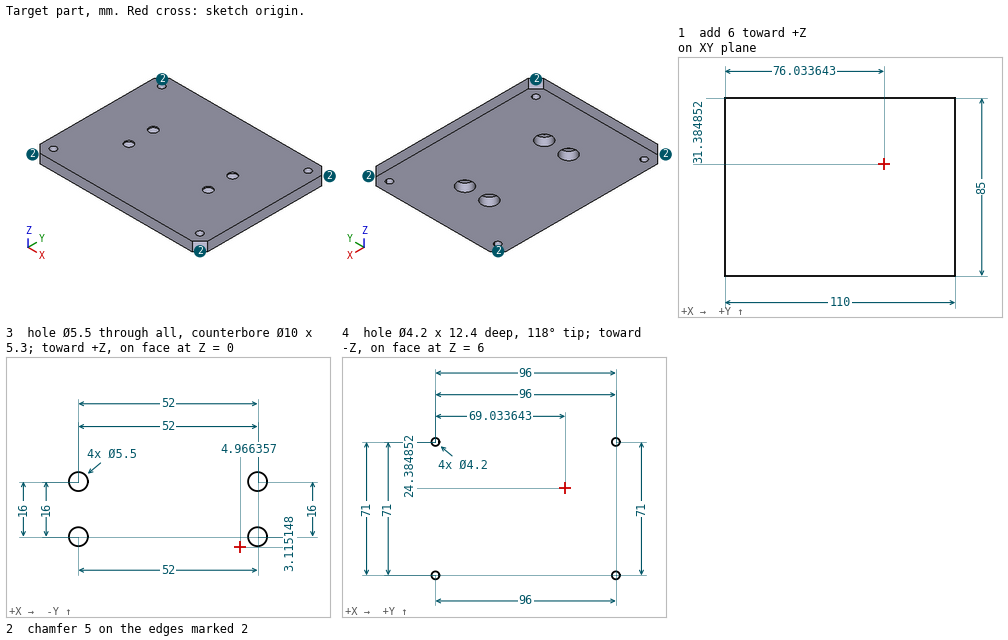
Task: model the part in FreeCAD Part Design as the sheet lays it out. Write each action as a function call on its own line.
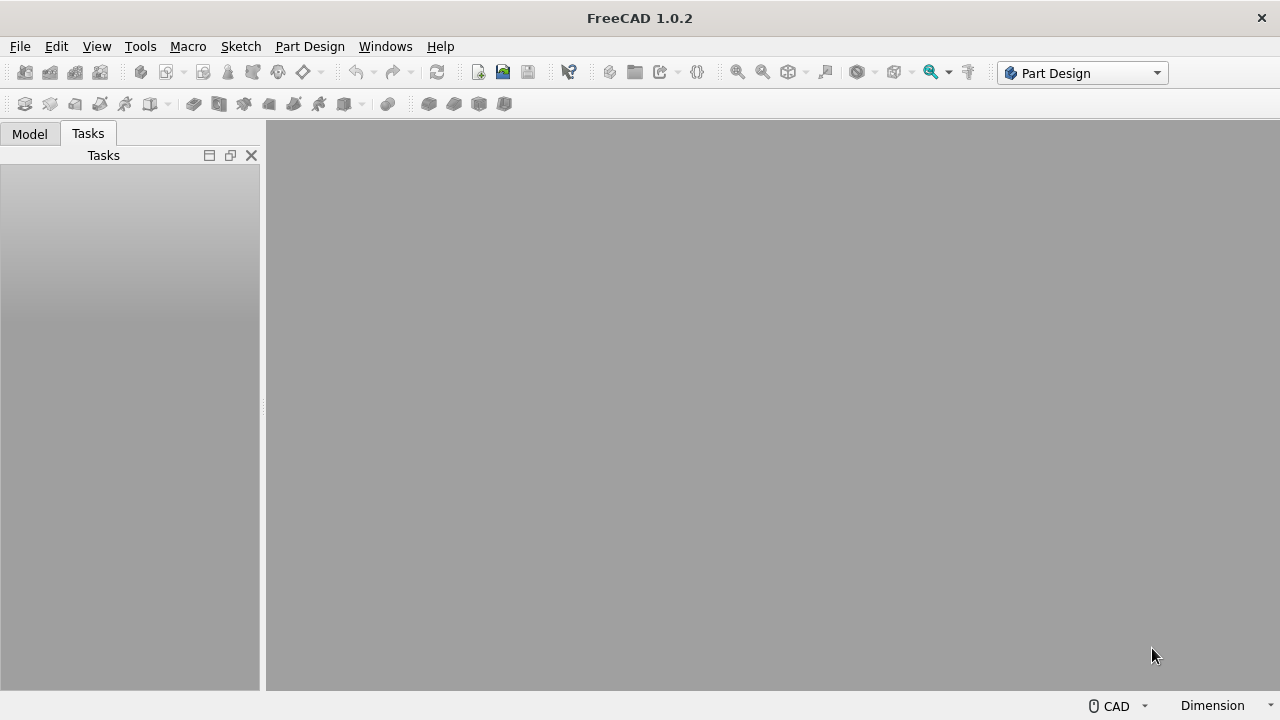
click(478, 72)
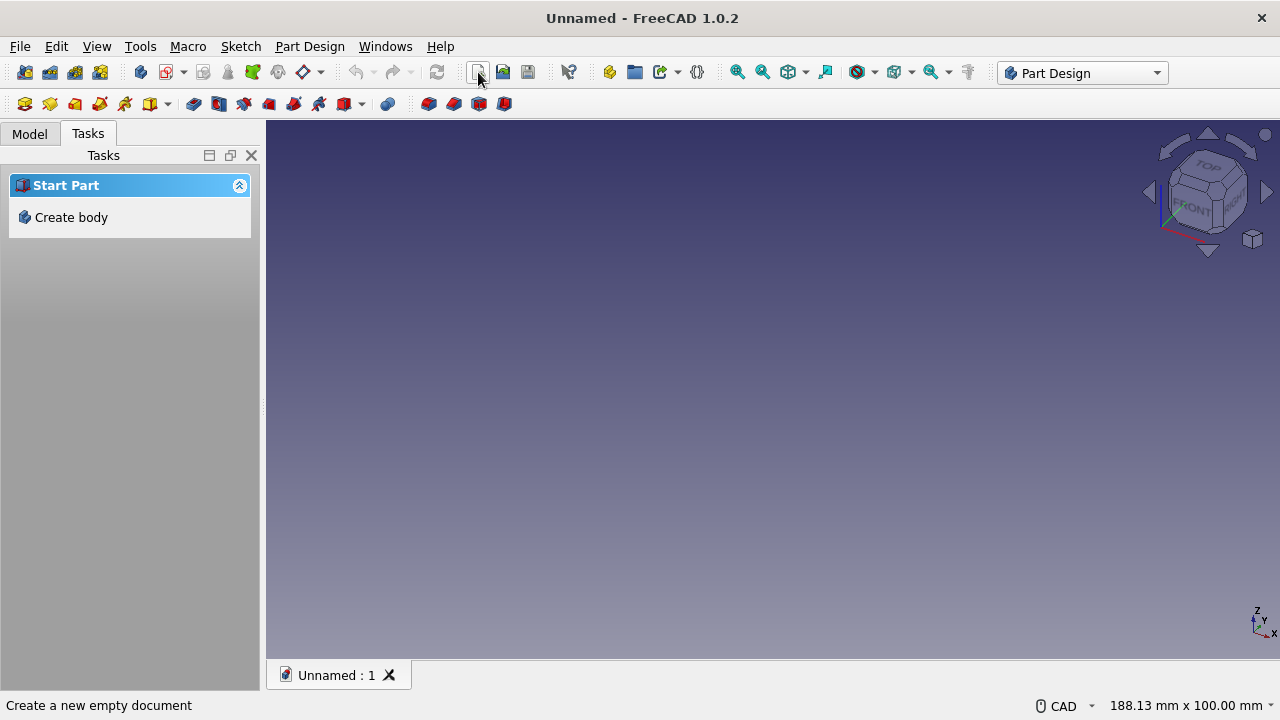
click(166, 72)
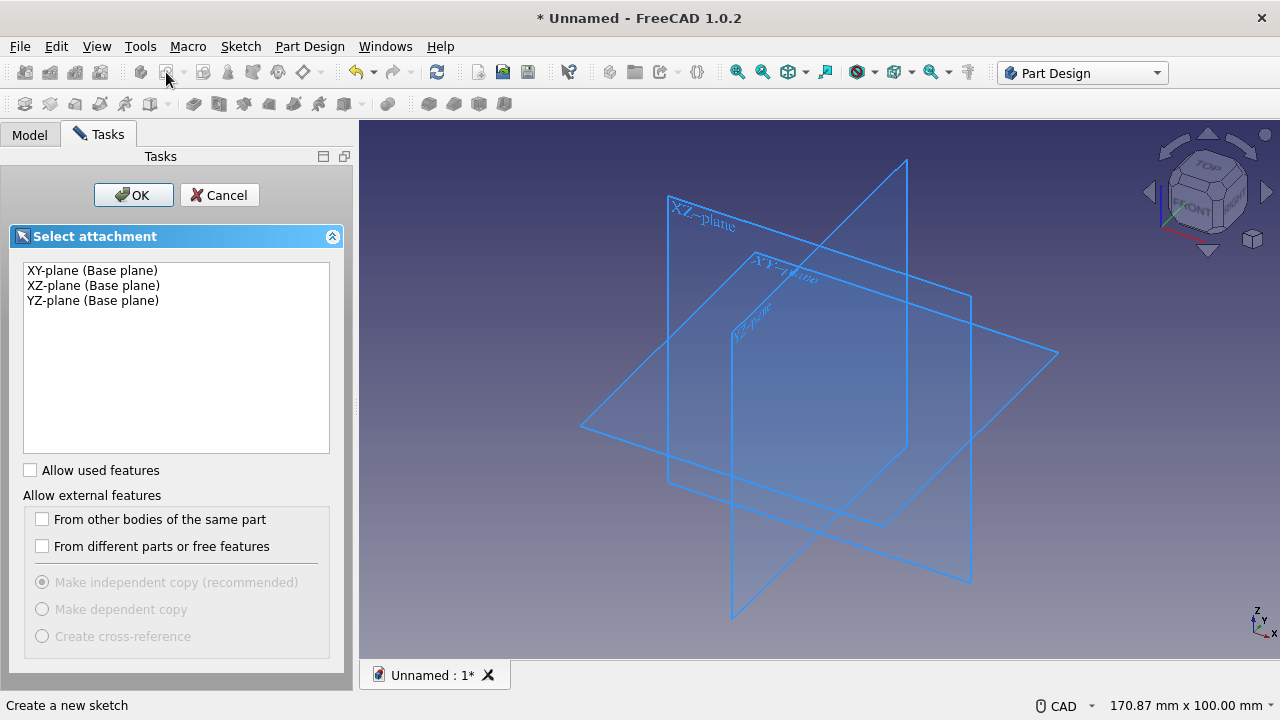
click(84, 270)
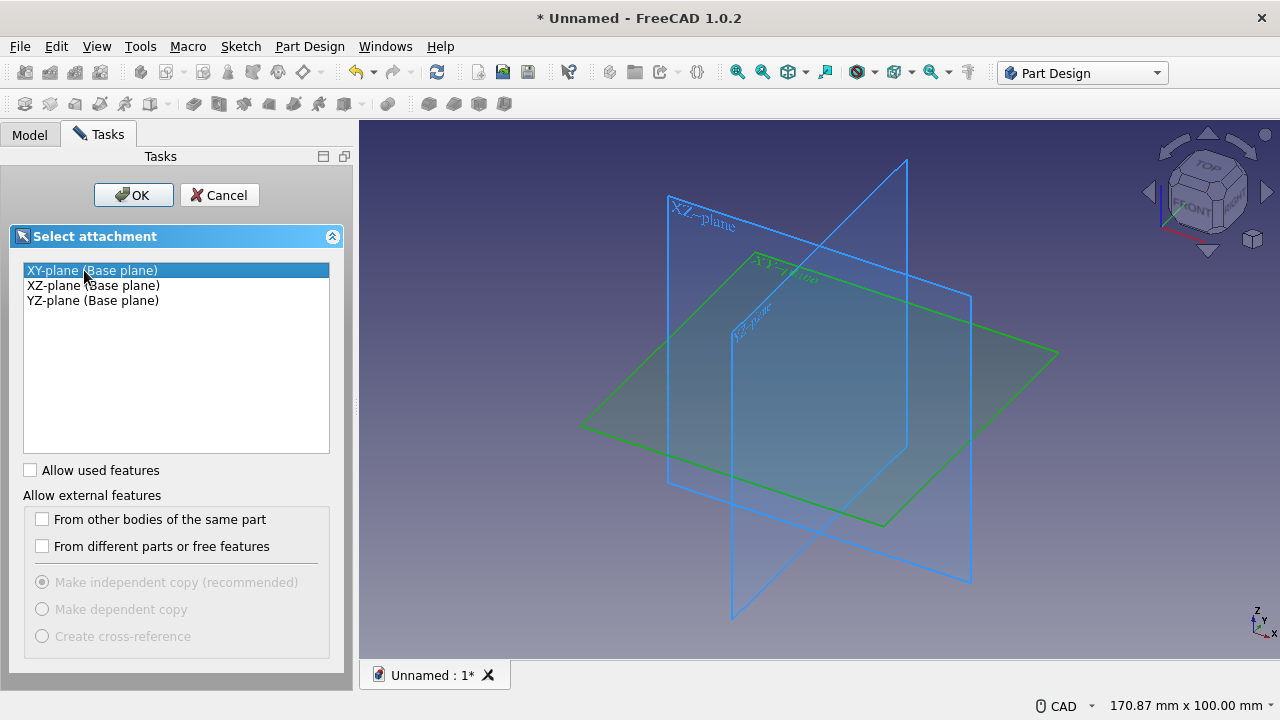
click(134, 195)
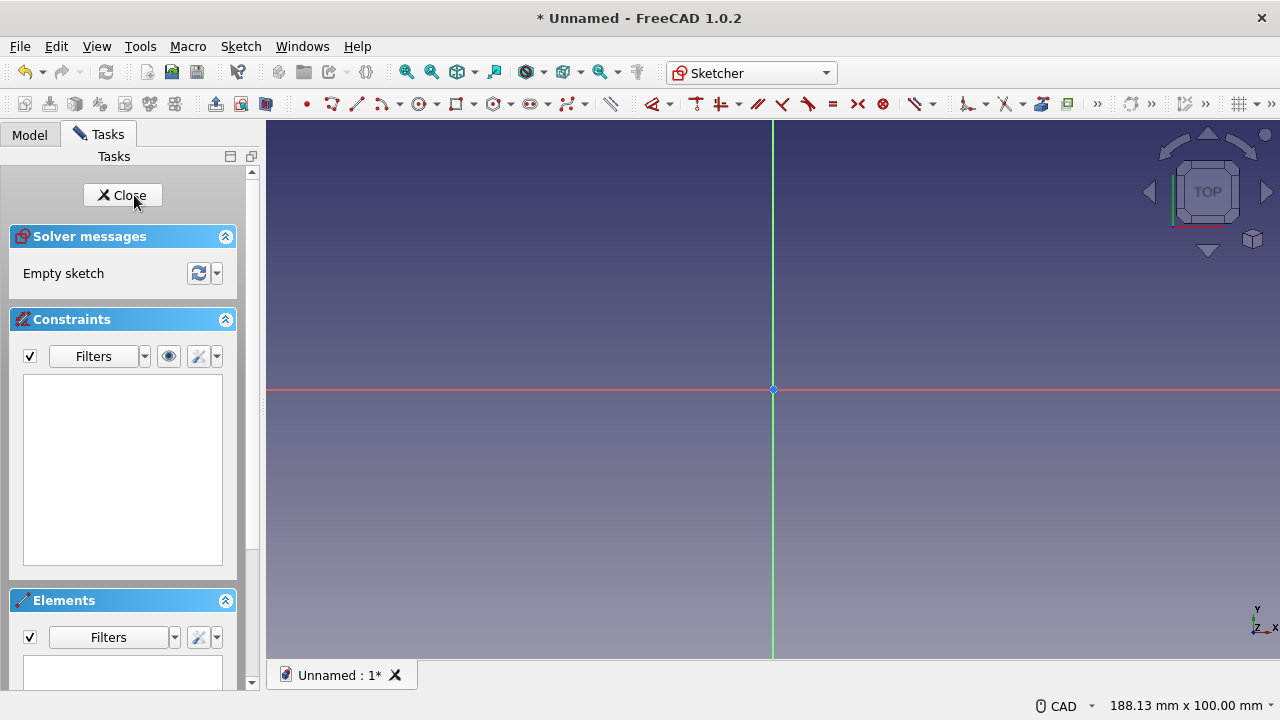
scroll(907, 148, down, 1)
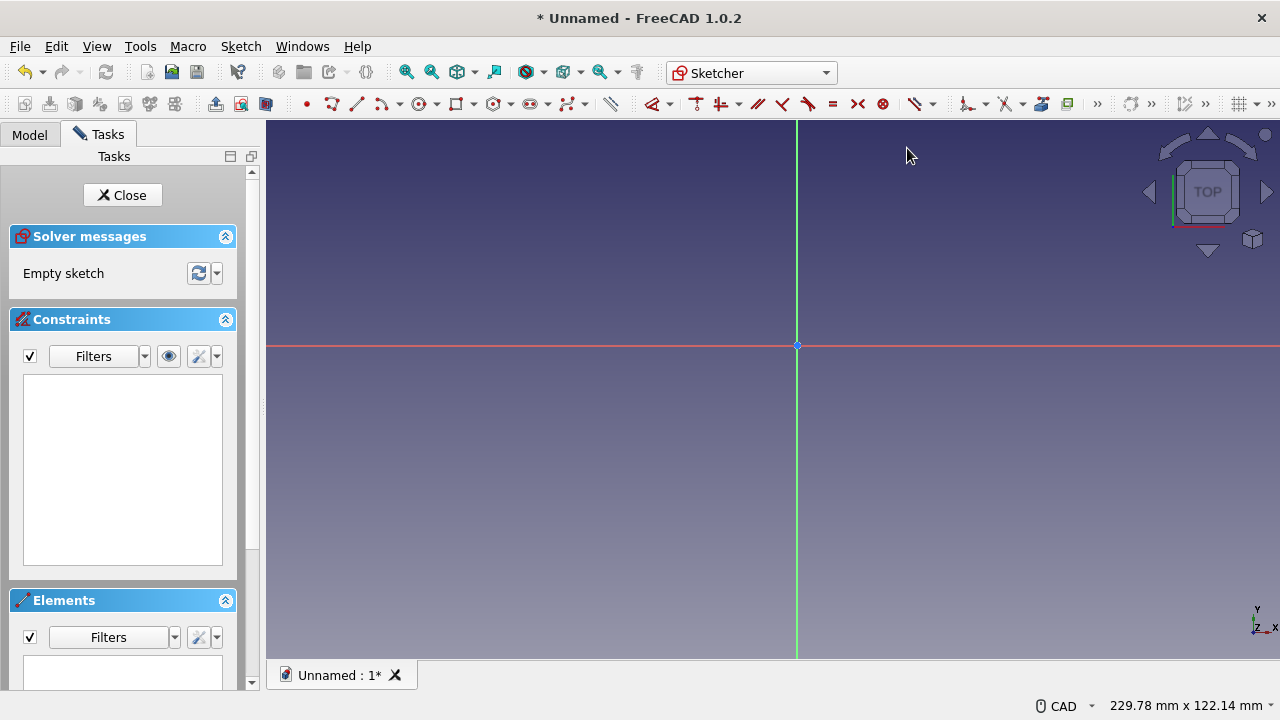
key(g)
key(r)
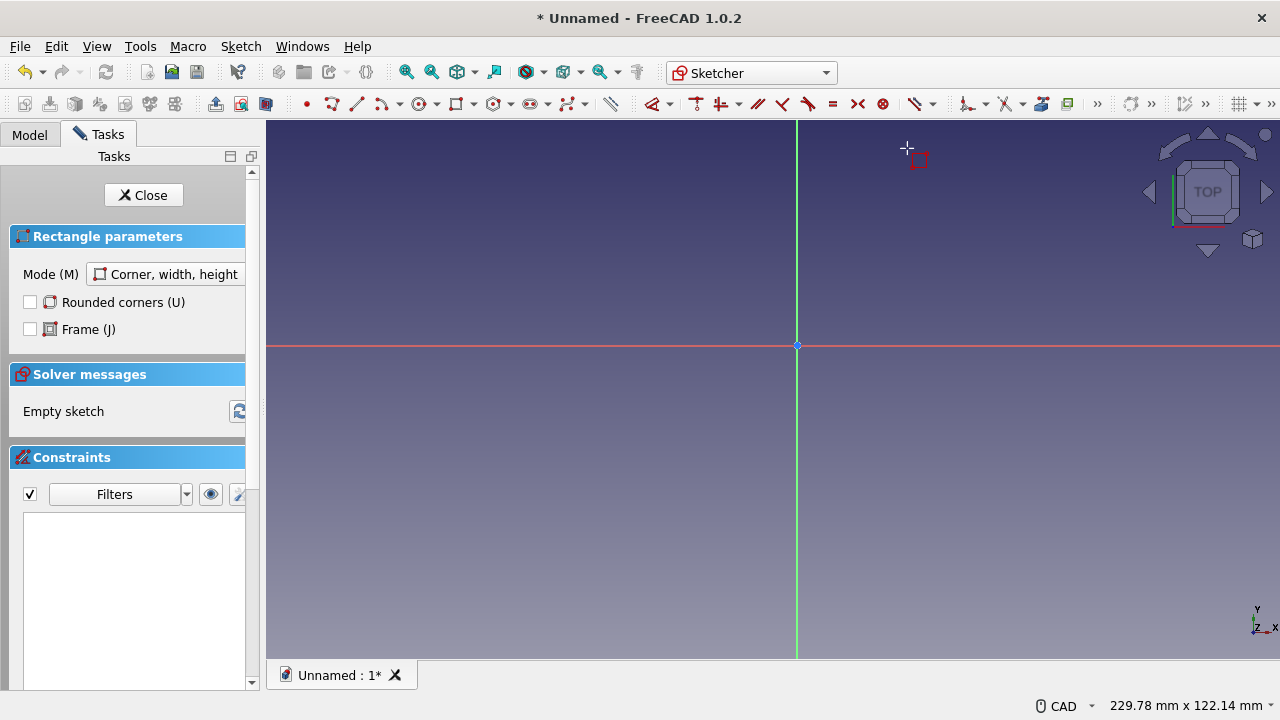
click(462, 207)
move(947, 582)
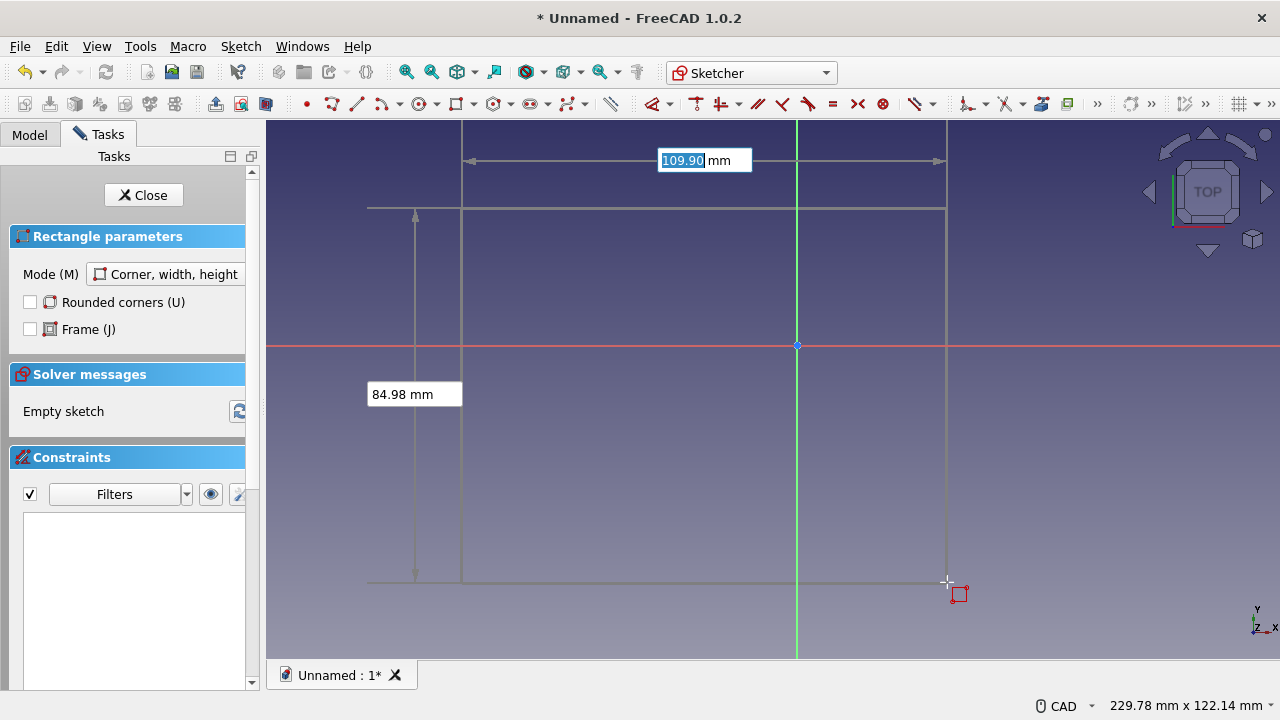
text(110)
key(Tab)
text(85)
key(Return)
key(Escape)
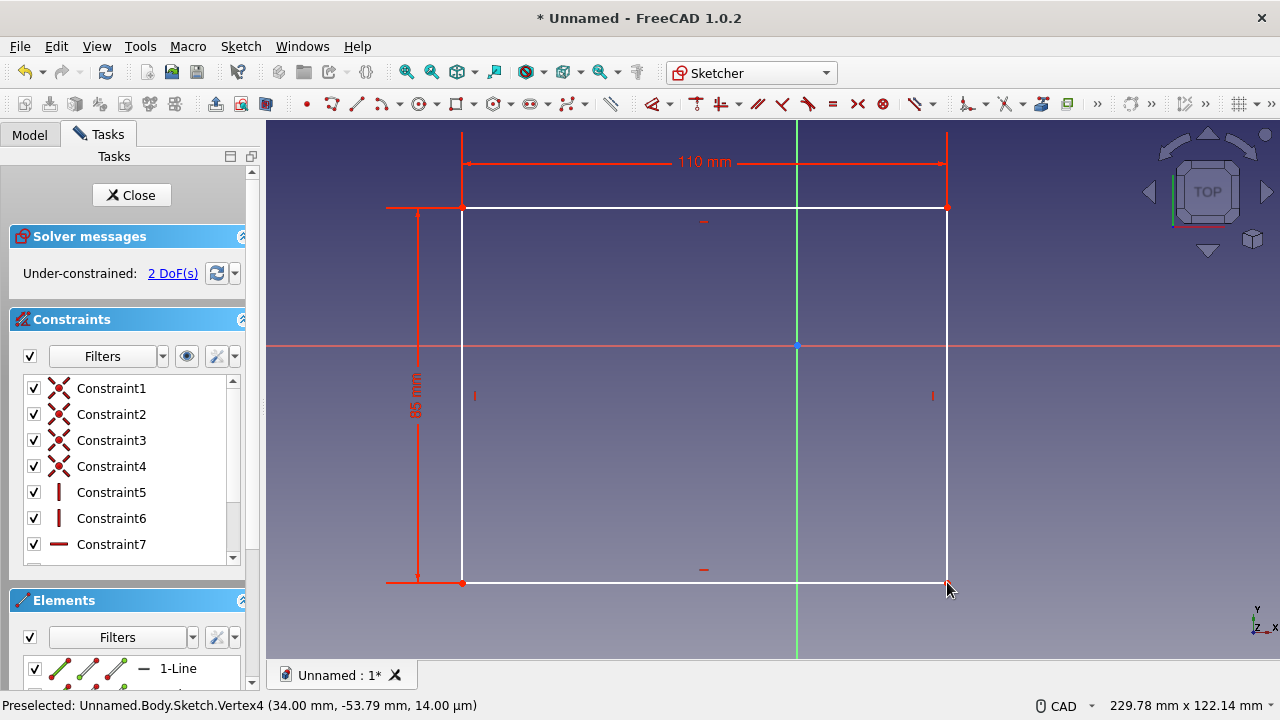
click(462, 208)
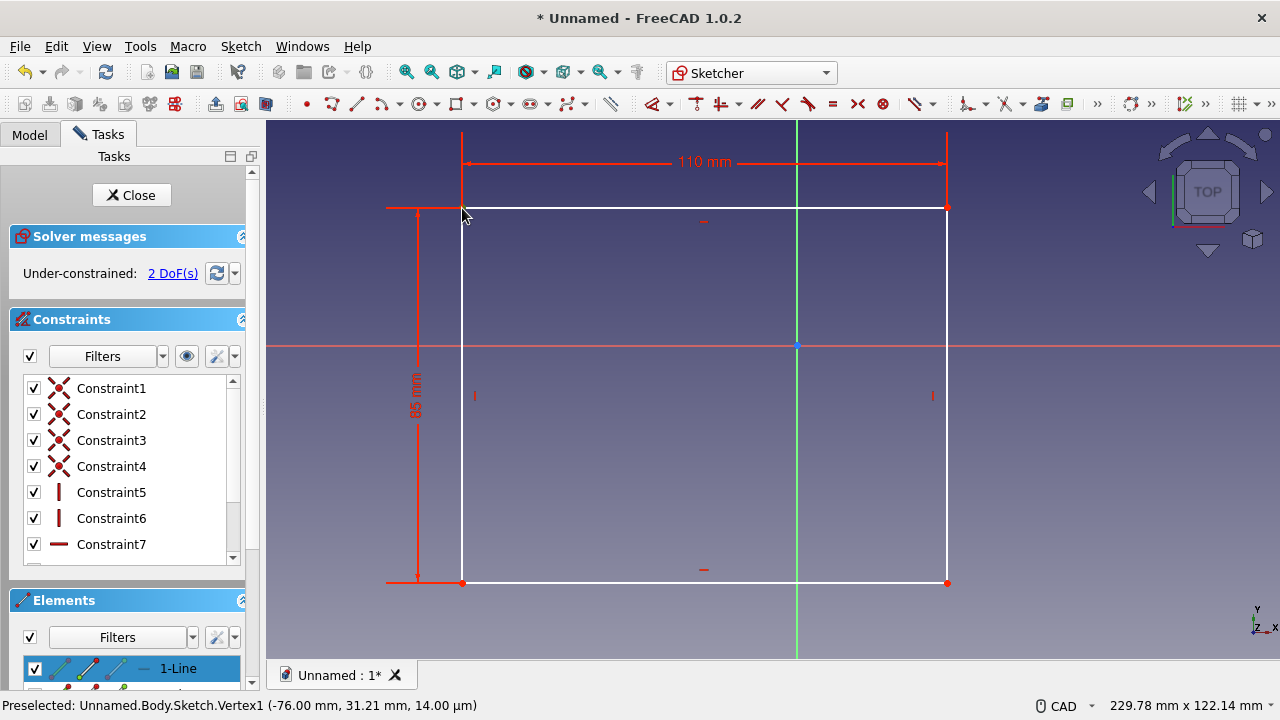
key(l)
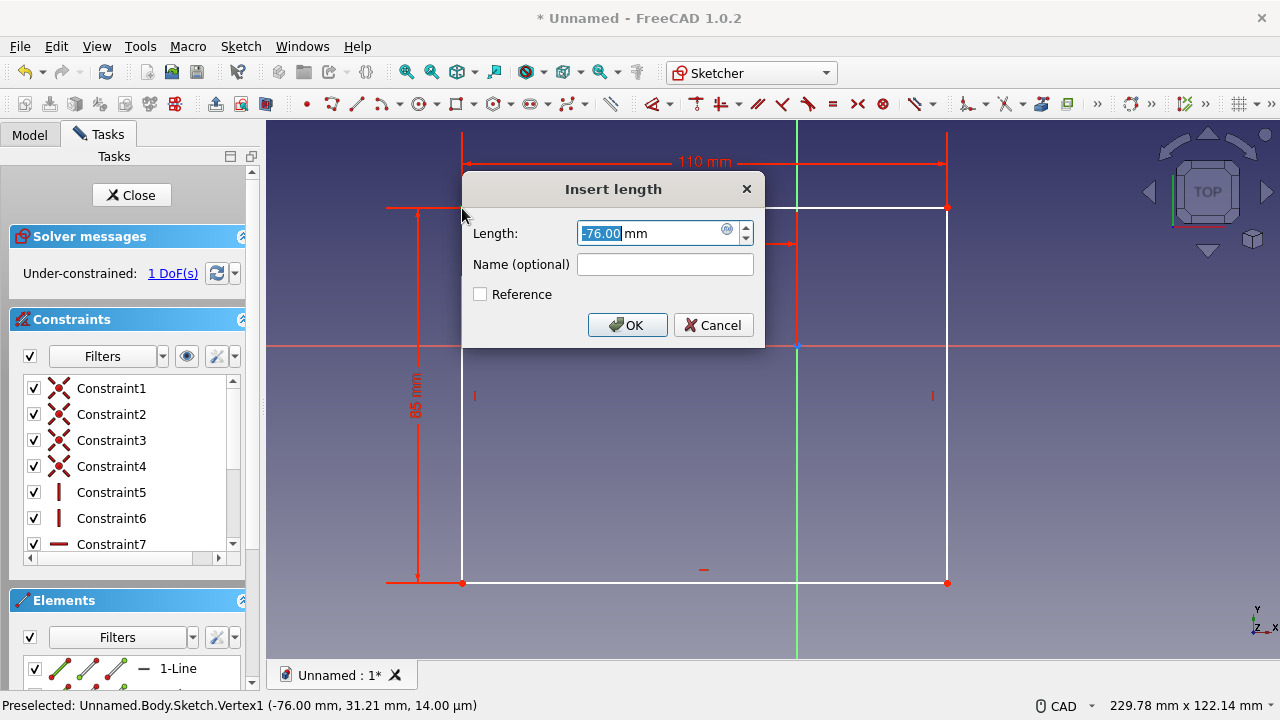
text(-76.033643)
key(Return)